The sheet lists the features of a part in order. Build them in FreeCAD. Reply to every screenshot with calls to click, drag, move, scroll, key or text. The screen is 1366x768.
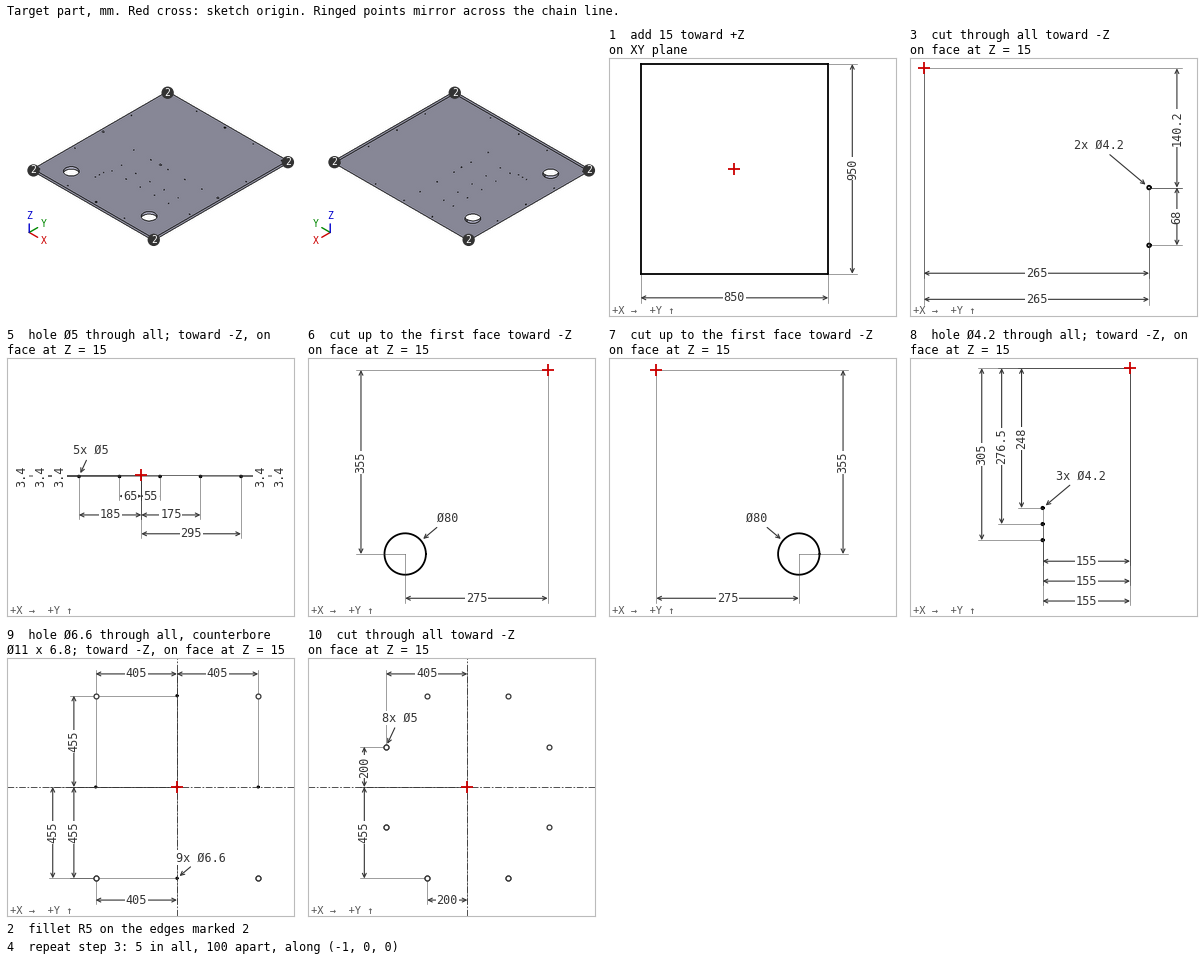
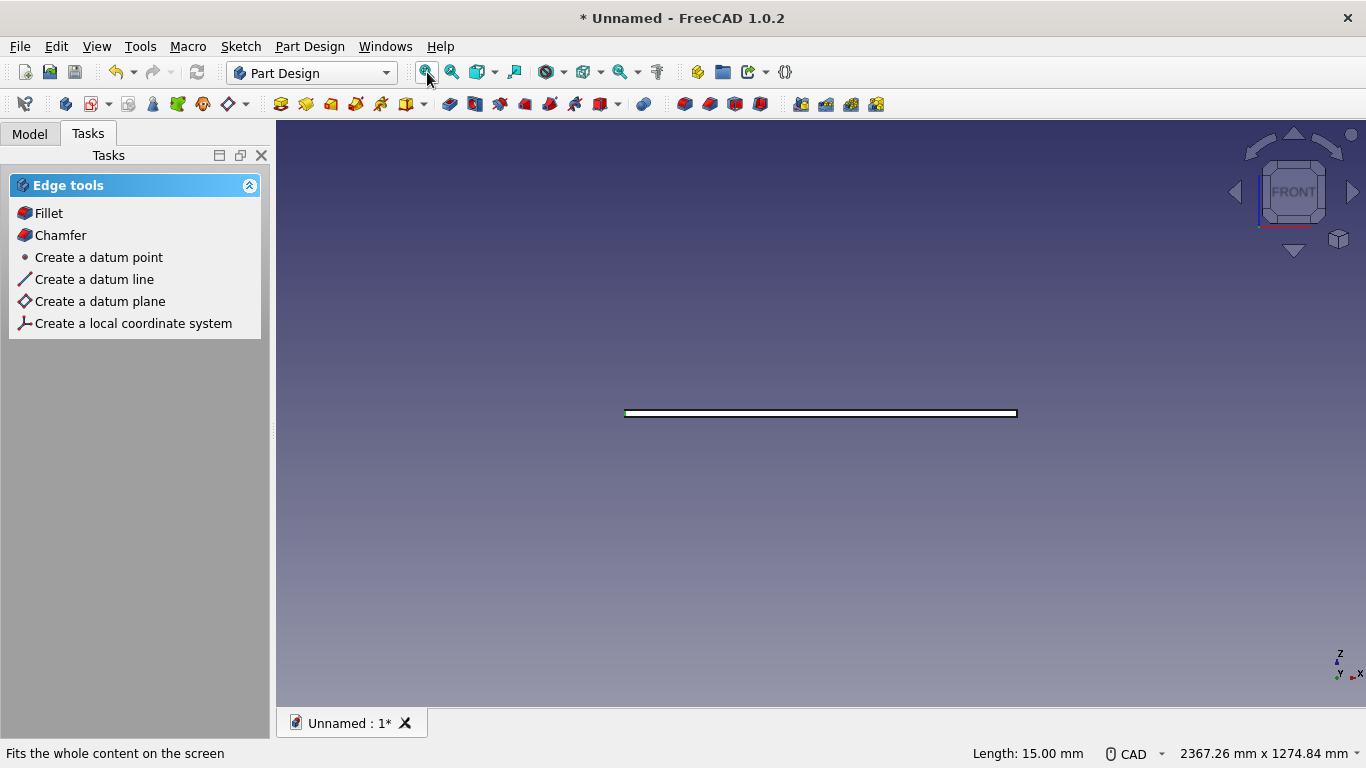
key(3)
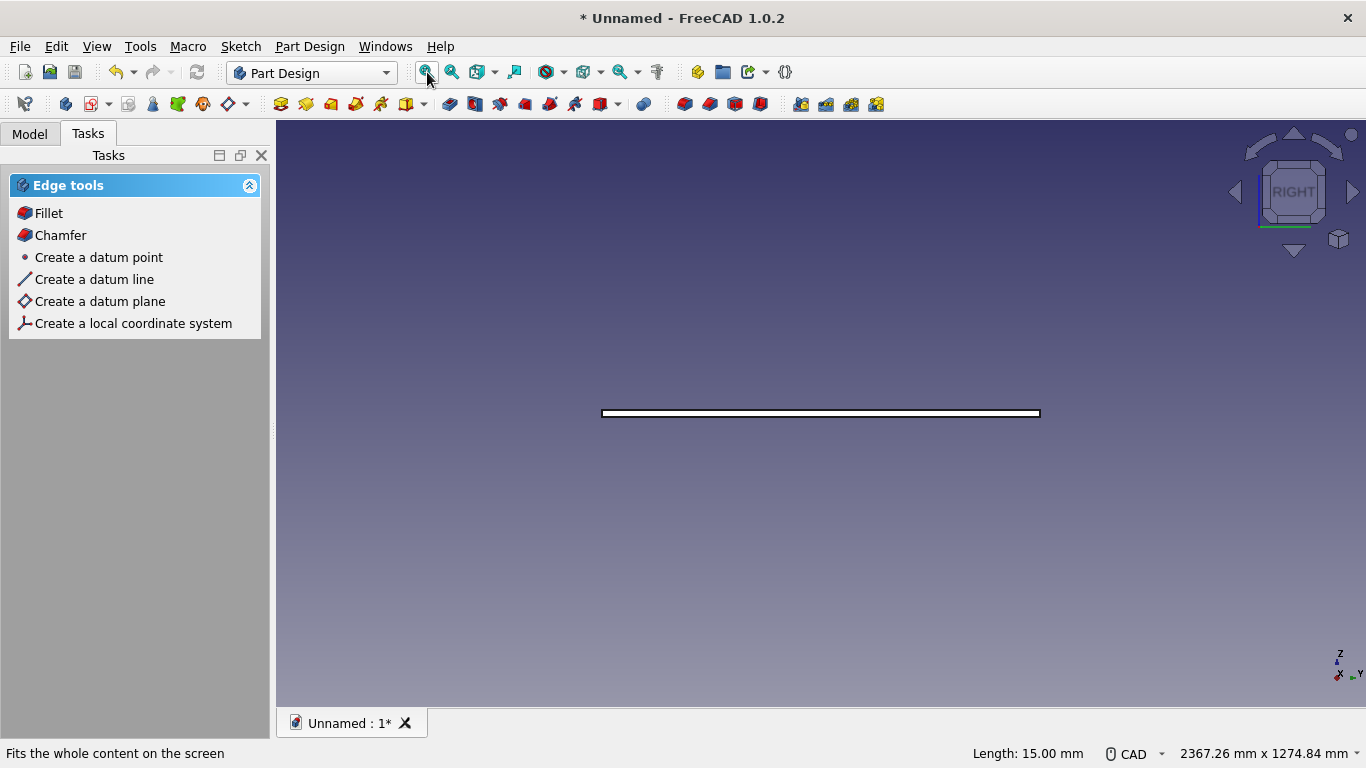
click(427, 72)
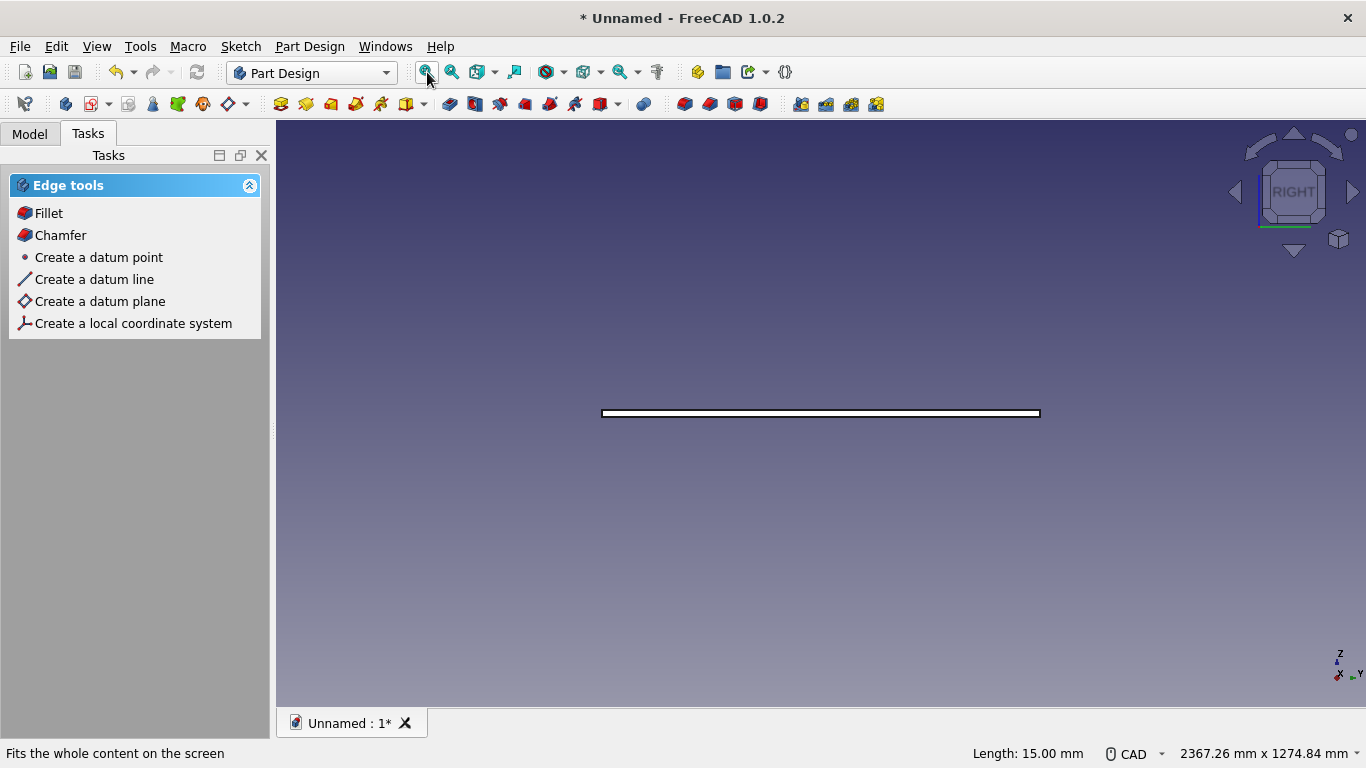
scroll(1040, 412, up, 9)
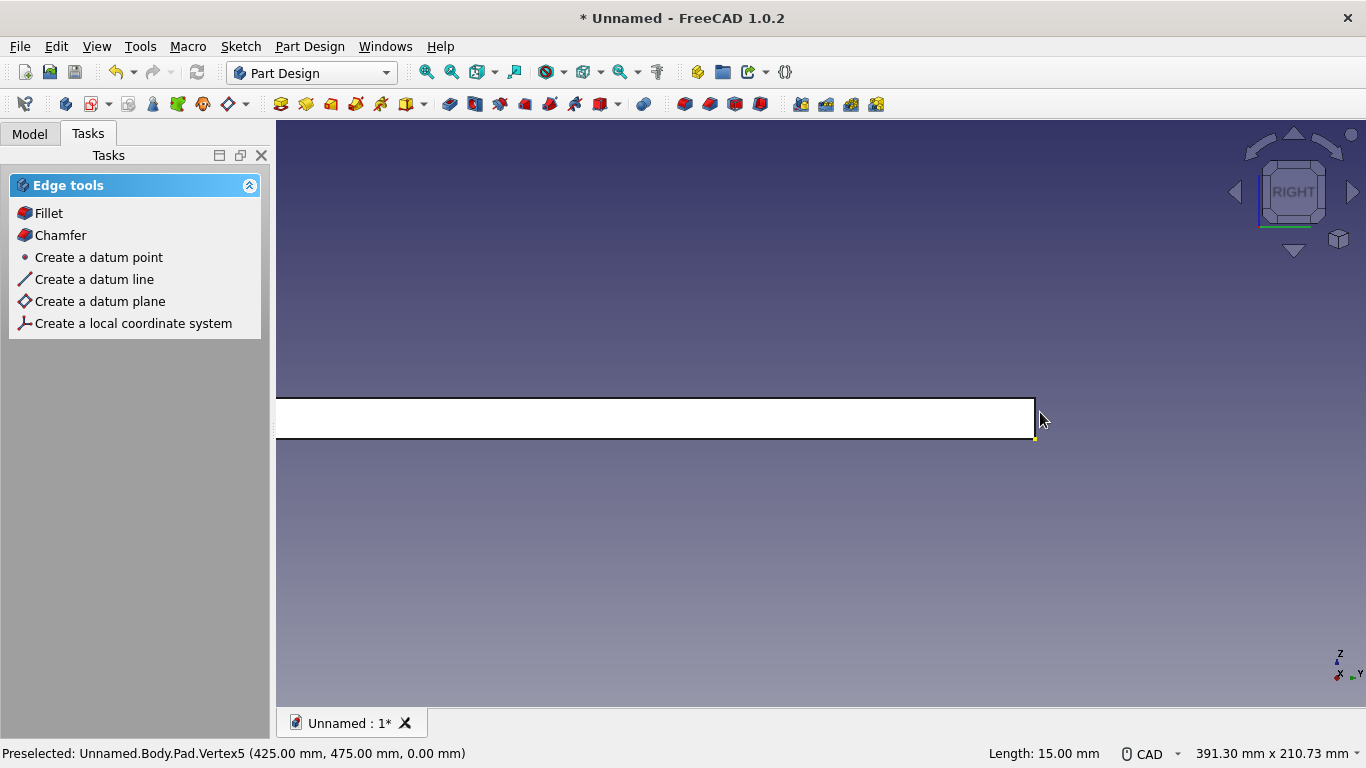
click(1035, 418, ctrl)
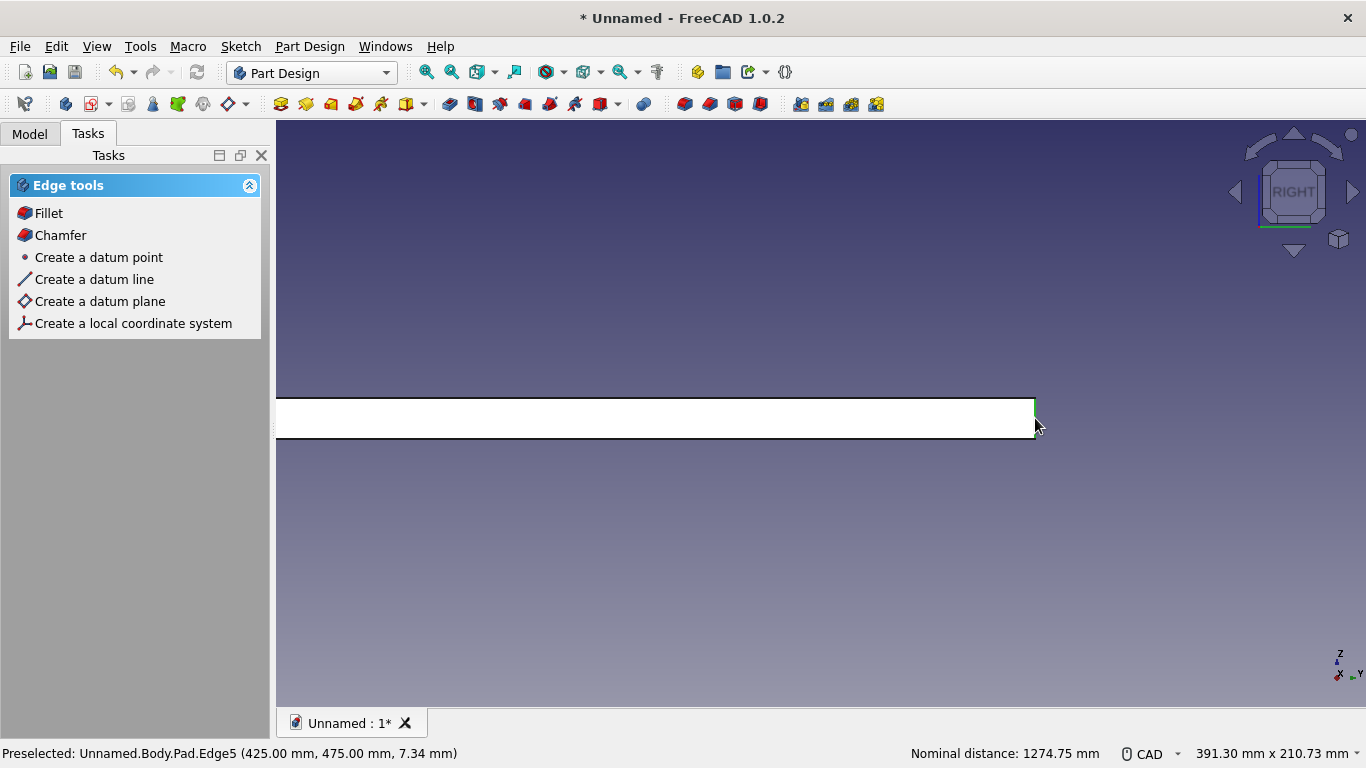
click(427, 72)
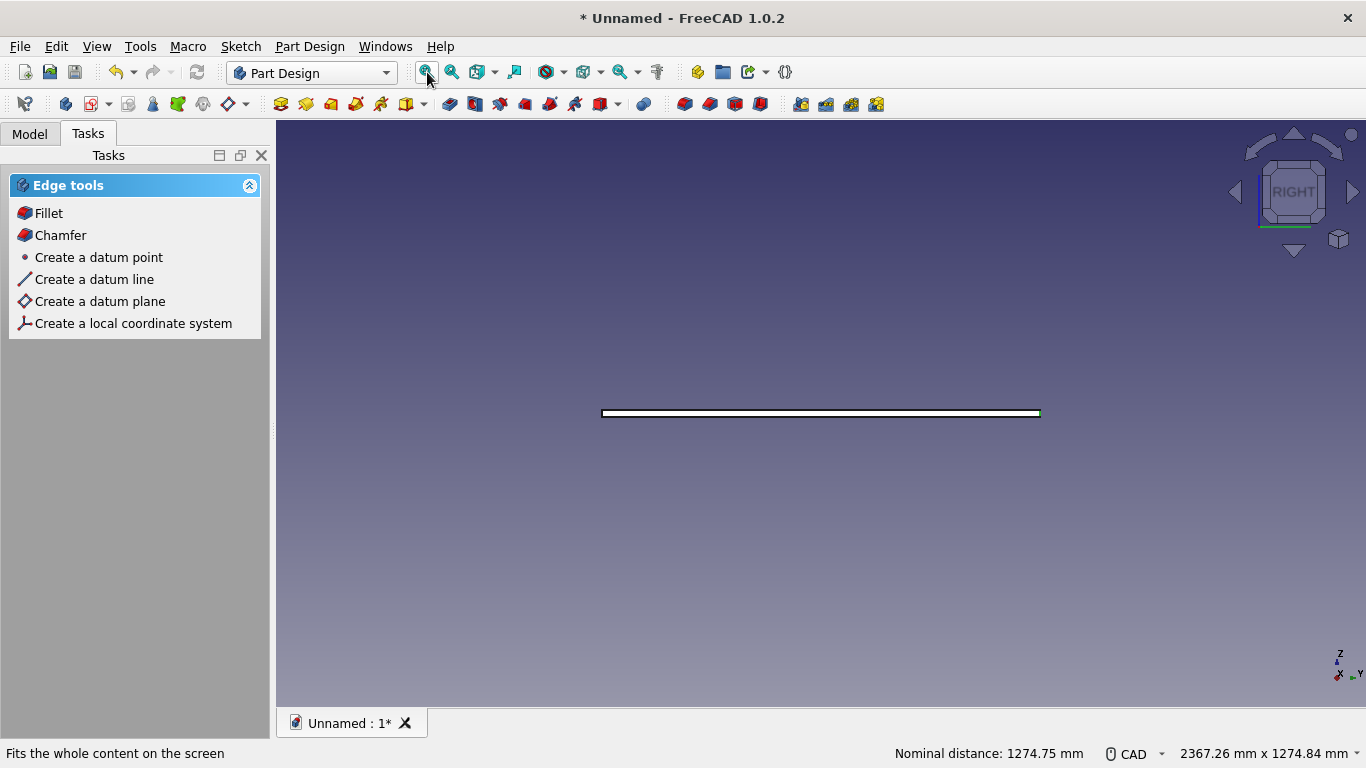
key(5)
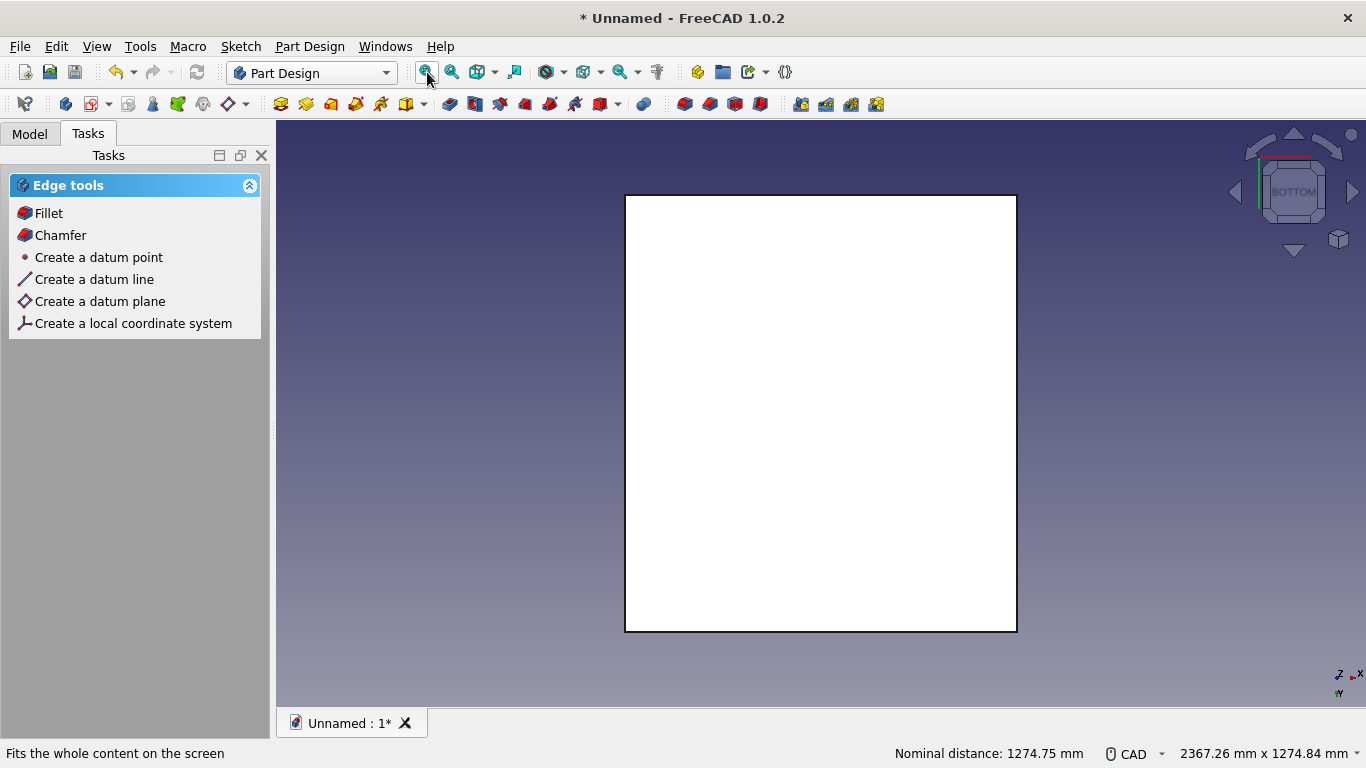
scroll(625, 631, up, 9)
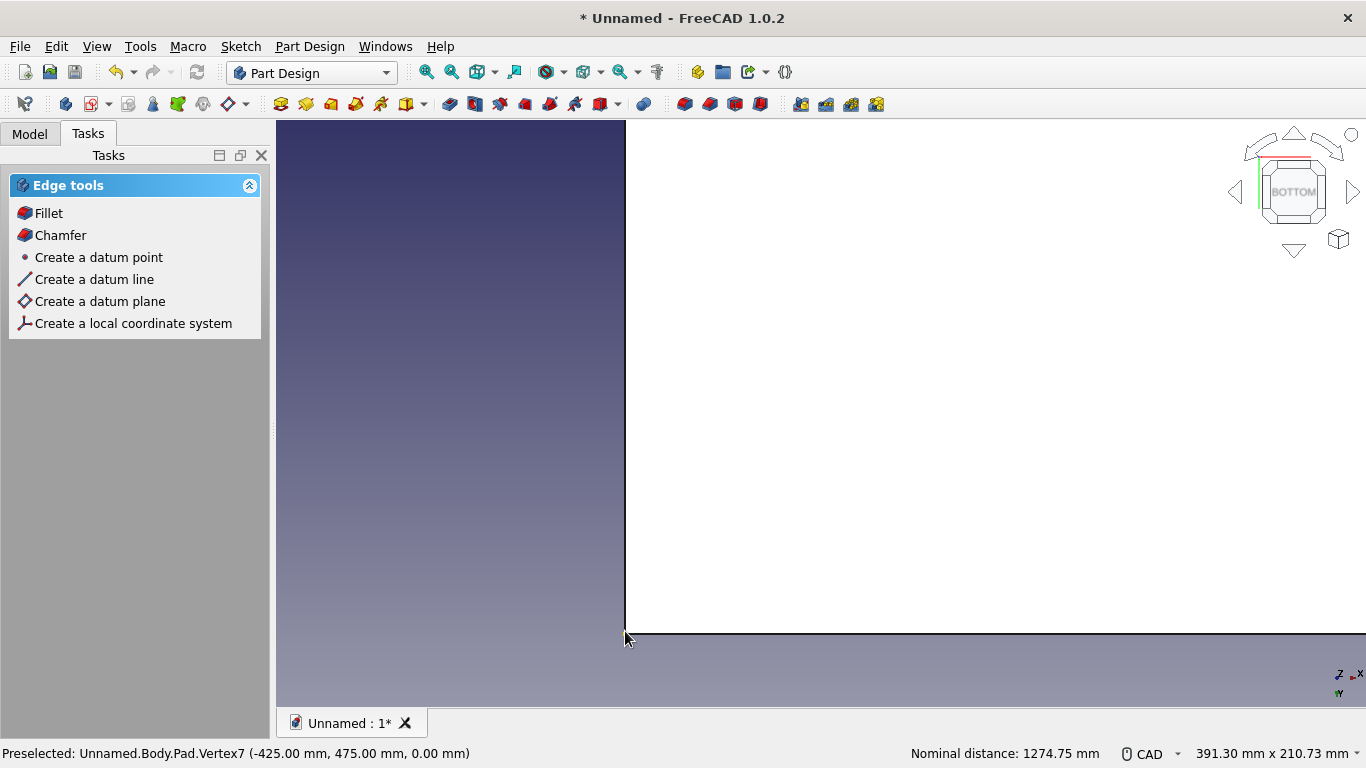
click(427, 72)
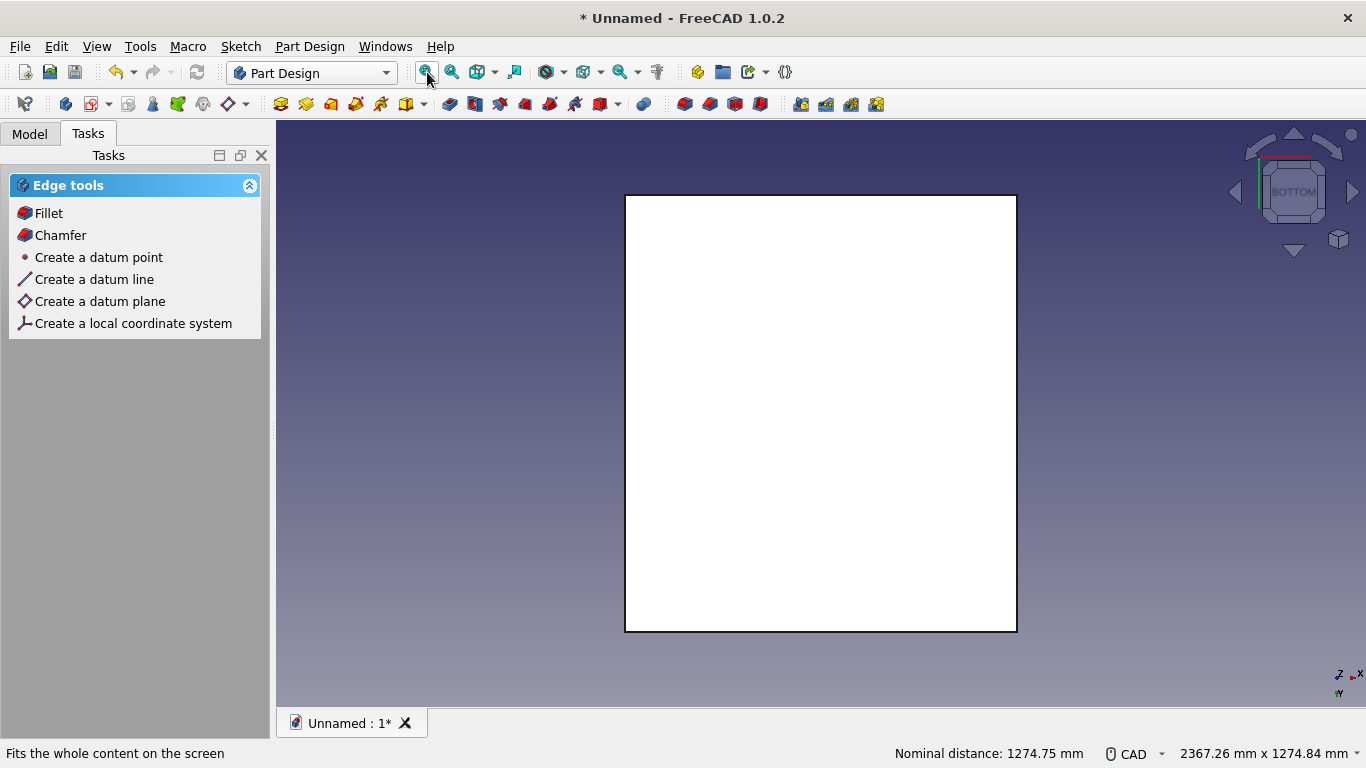
key(4)